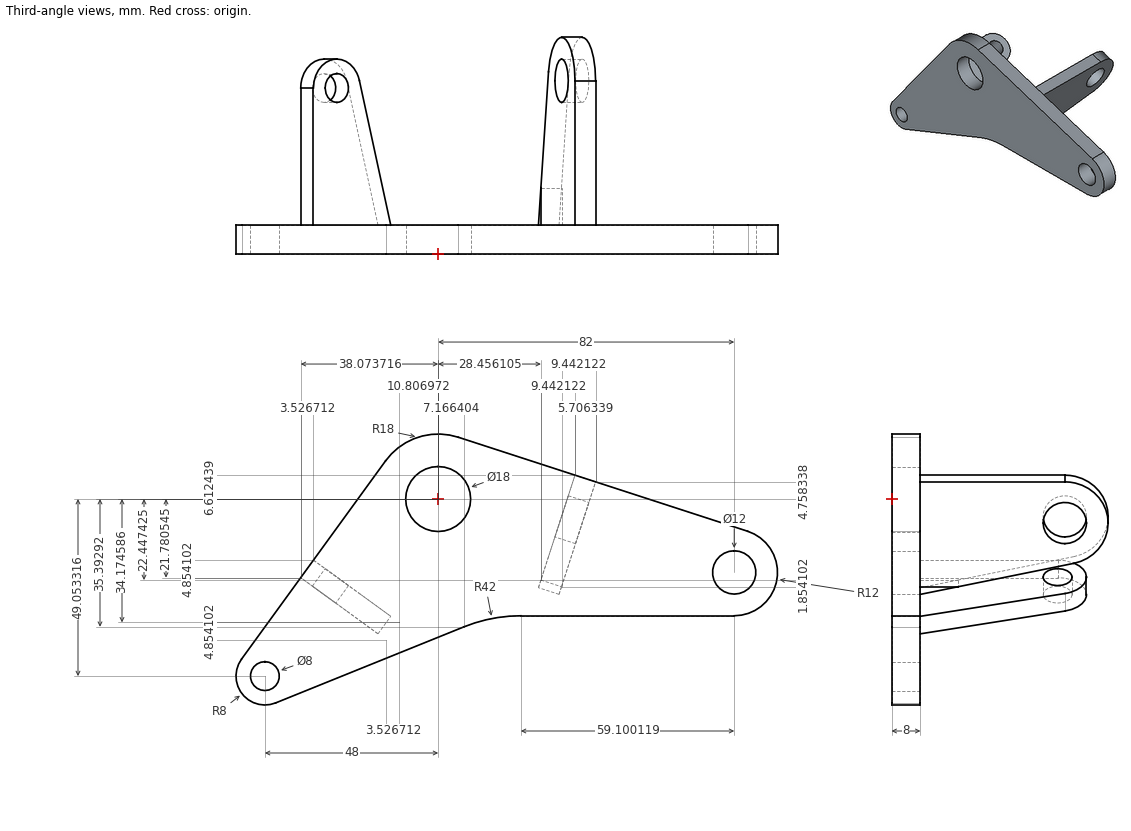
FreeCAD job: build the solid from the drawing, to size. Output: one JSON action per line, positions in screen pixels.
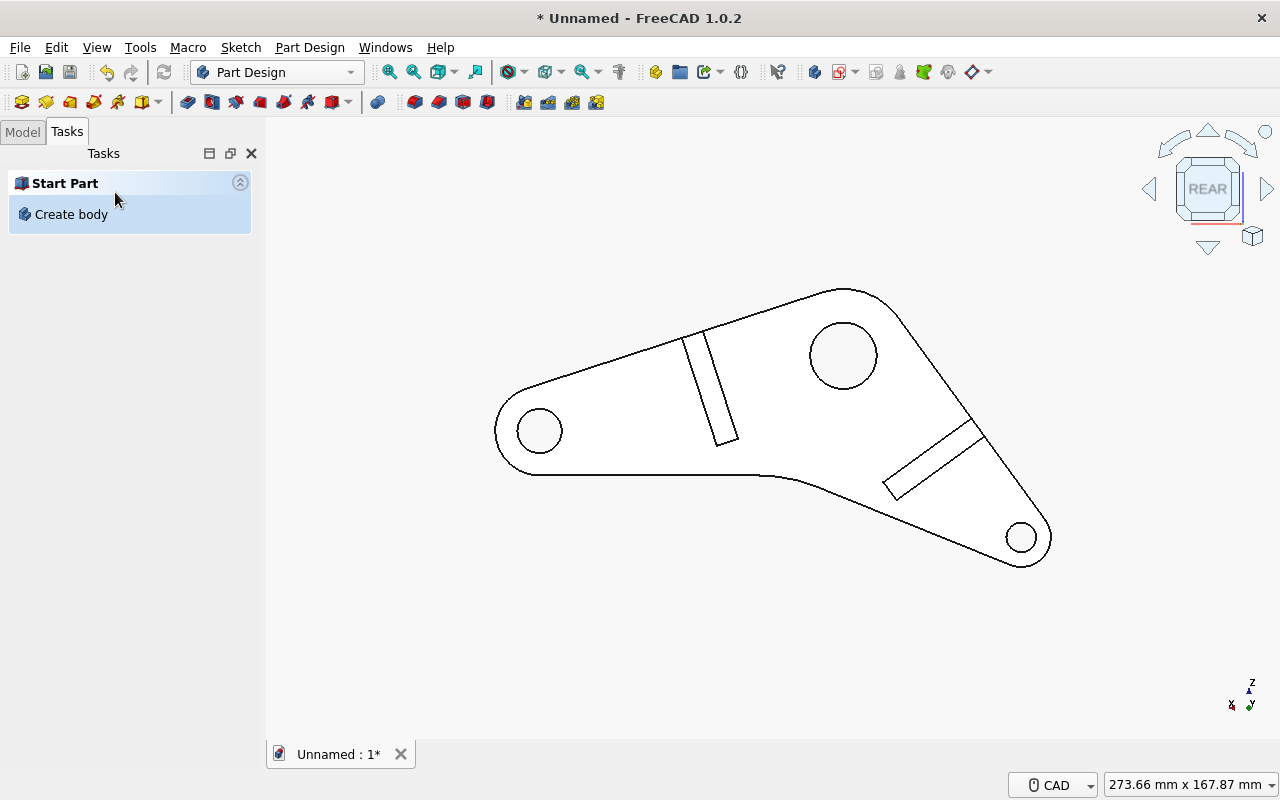
{"action": "key", "text": "5"}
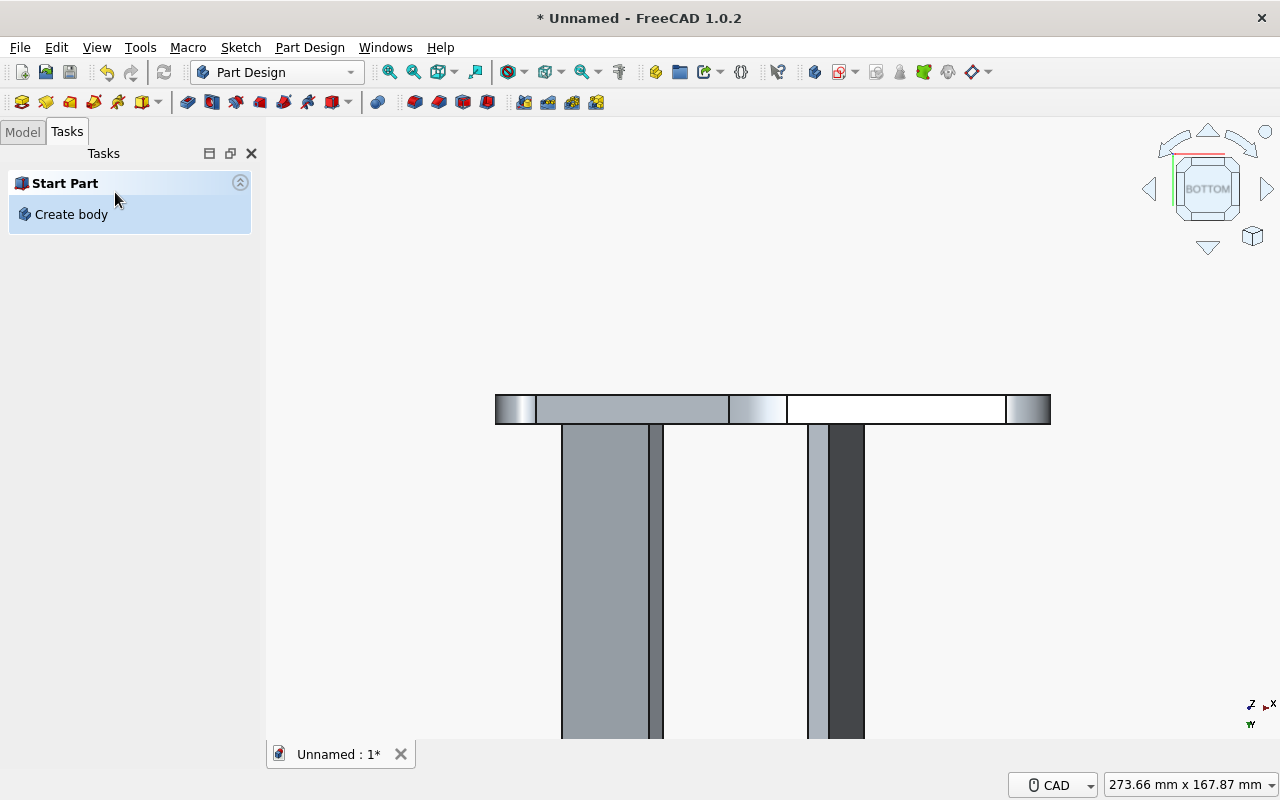
{"action": "key", "text": "v f"}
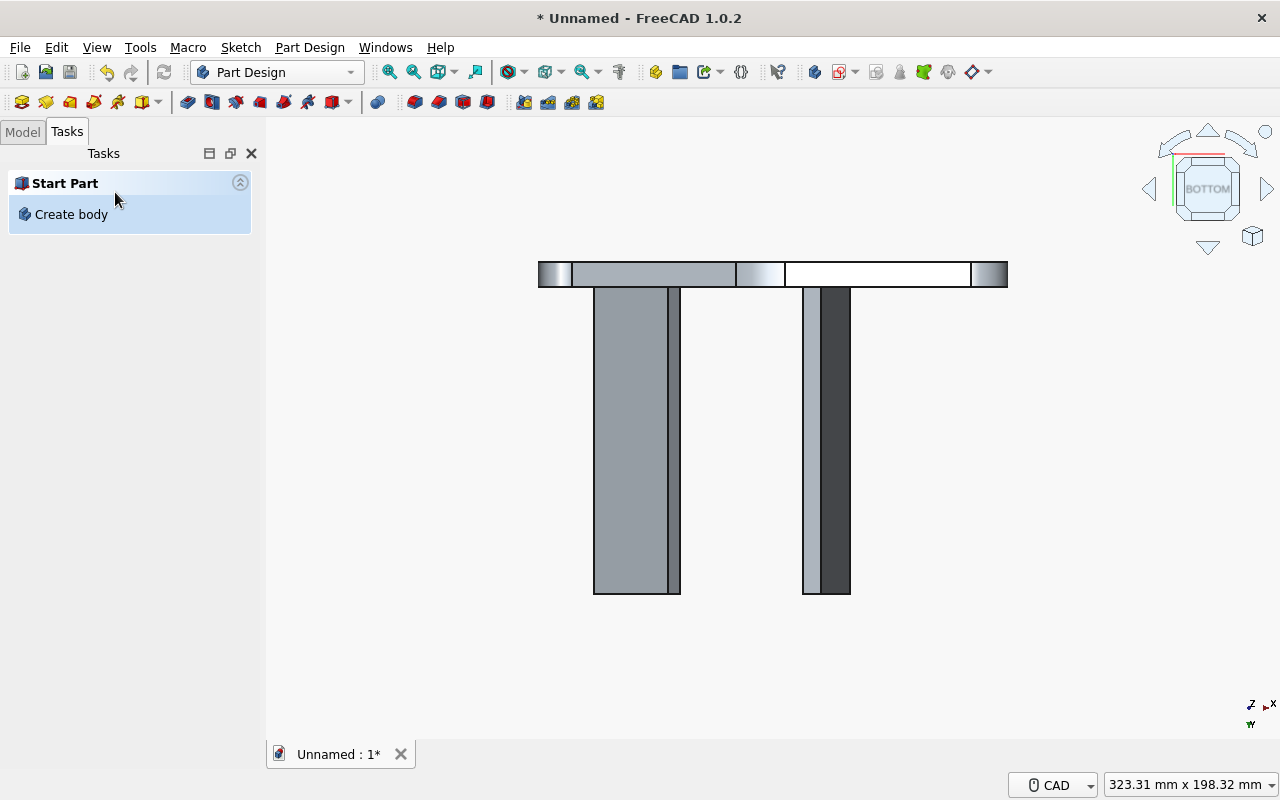
{"action": "left_click", "coordinate": [631, 527]}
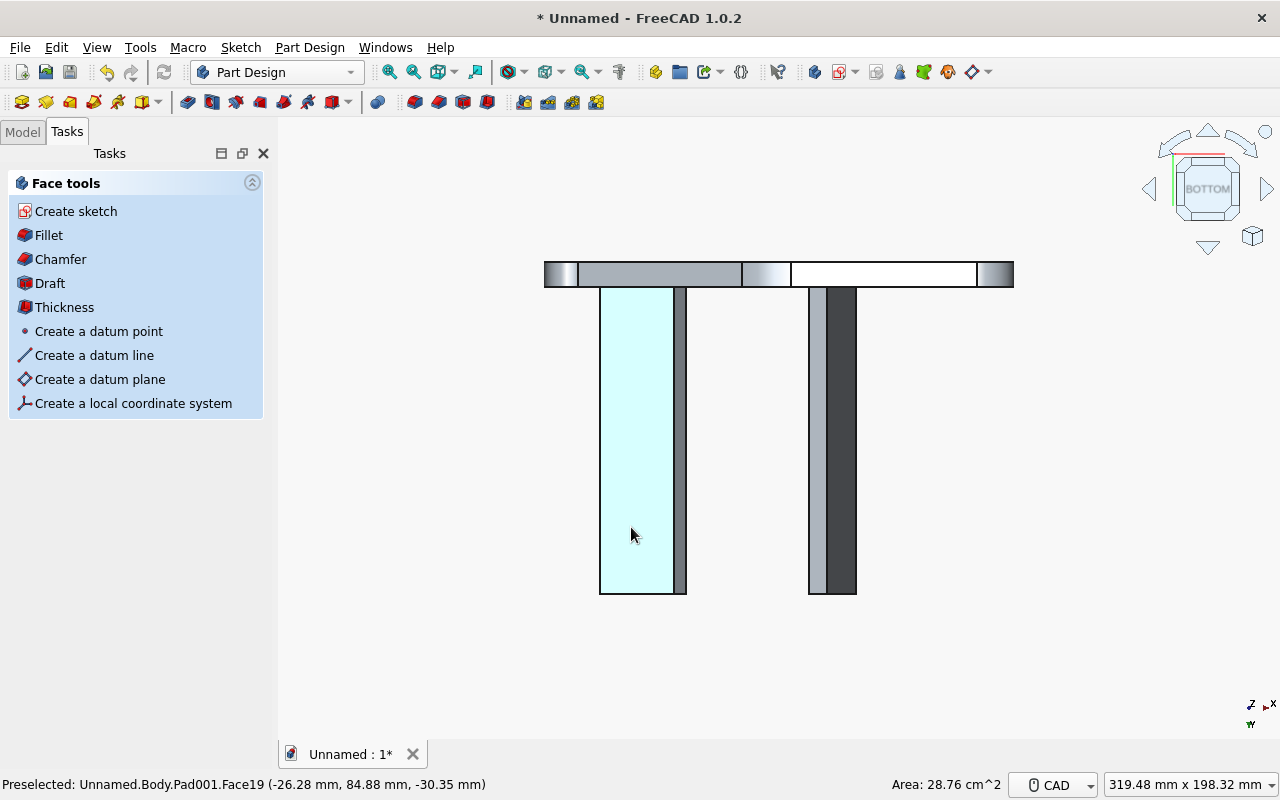
{"action": "left_click", "coordinate": [840, 72]}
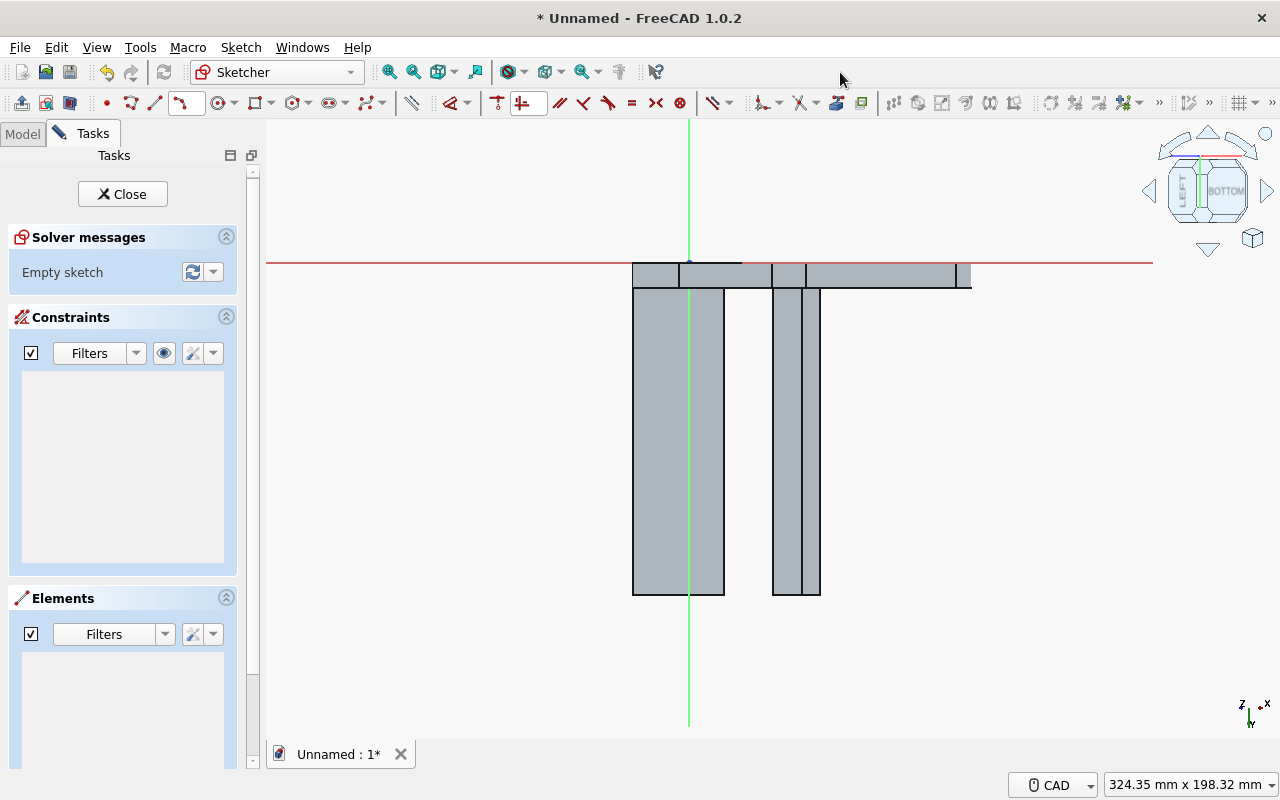
{"action": "left_click", "coordinate": [70, 104]}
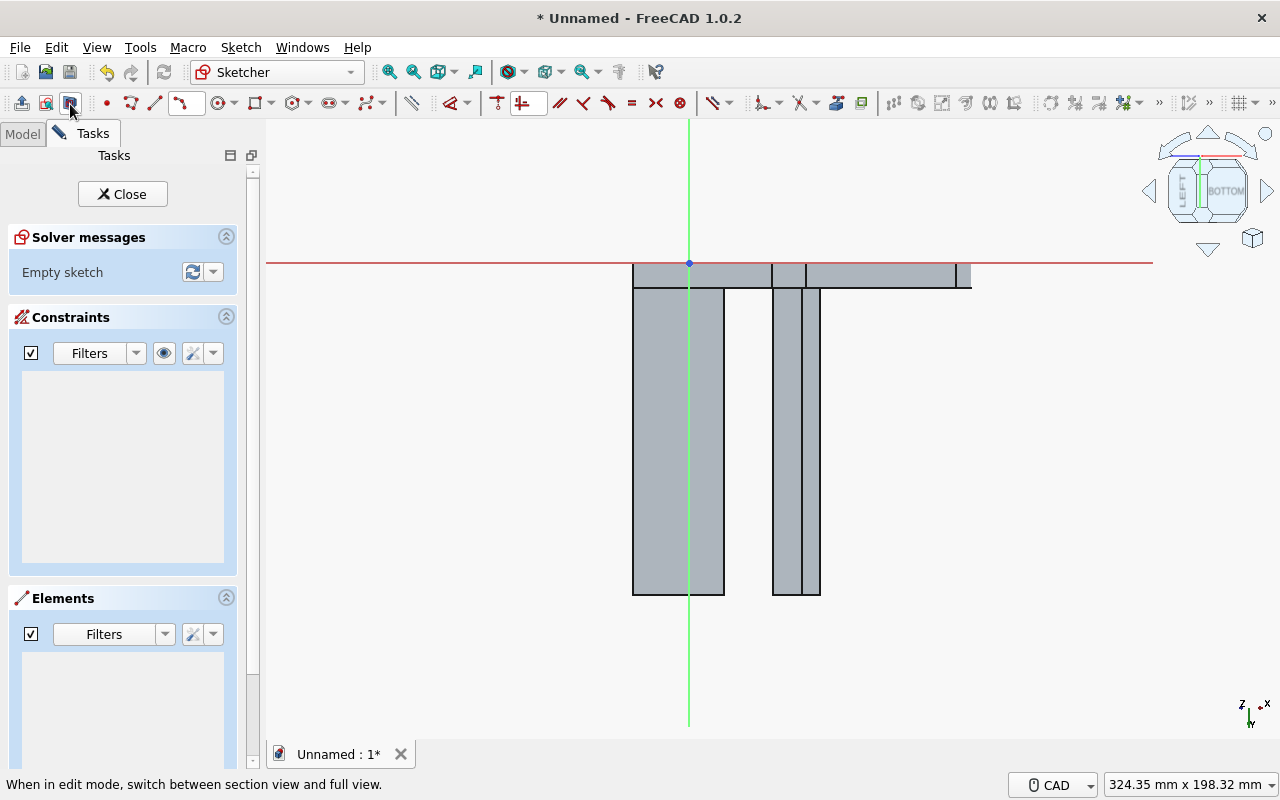
{"action": "left_click", "coordinate": [132, 104]}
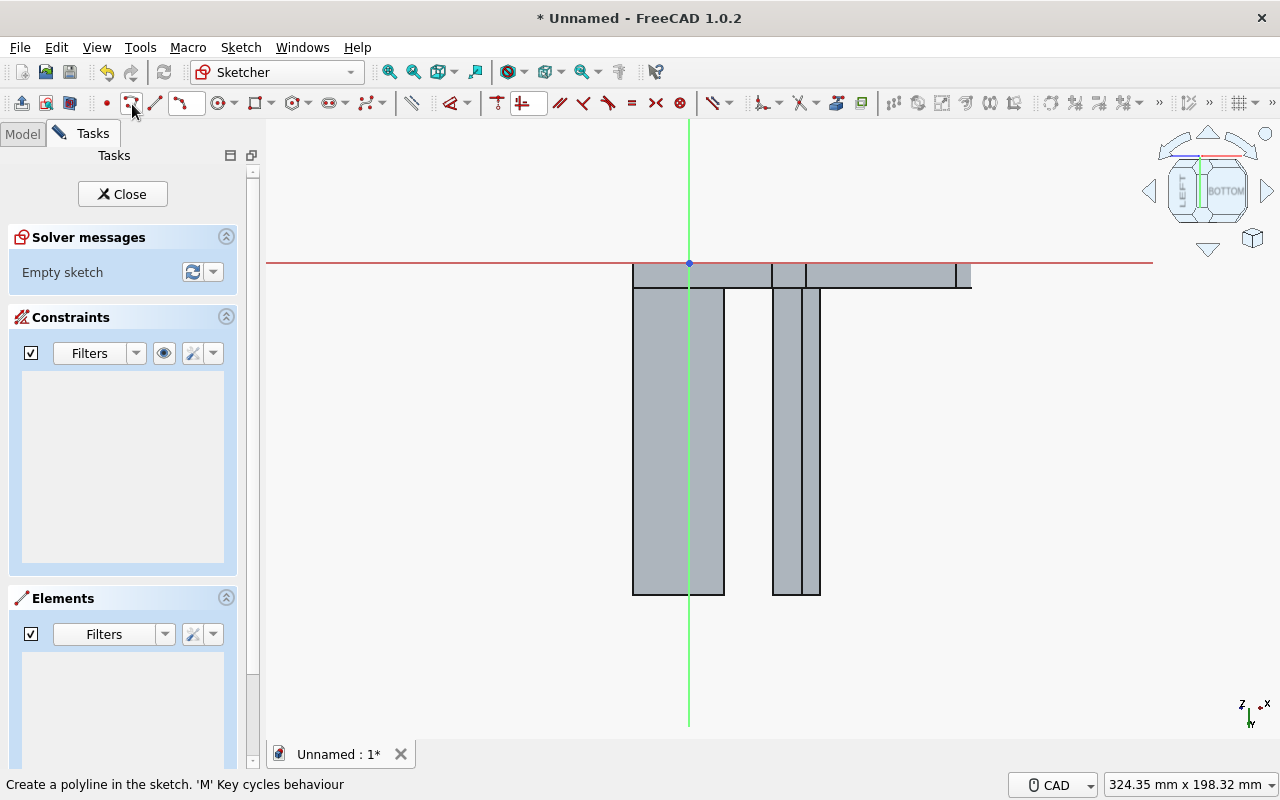
{"action": "left_click", "coordinate": [633, 407]}
{"action": "left_click", "coordinate": [614, 399]}
{"action": "left_click", "coordinate": [538, 609]}
{"action": "left_click", "coordinate": [746, 609]}
{"action": "left_click", "coordinate": [730, 288]}
{"action": "left_click", "coordinate": [715, 288]}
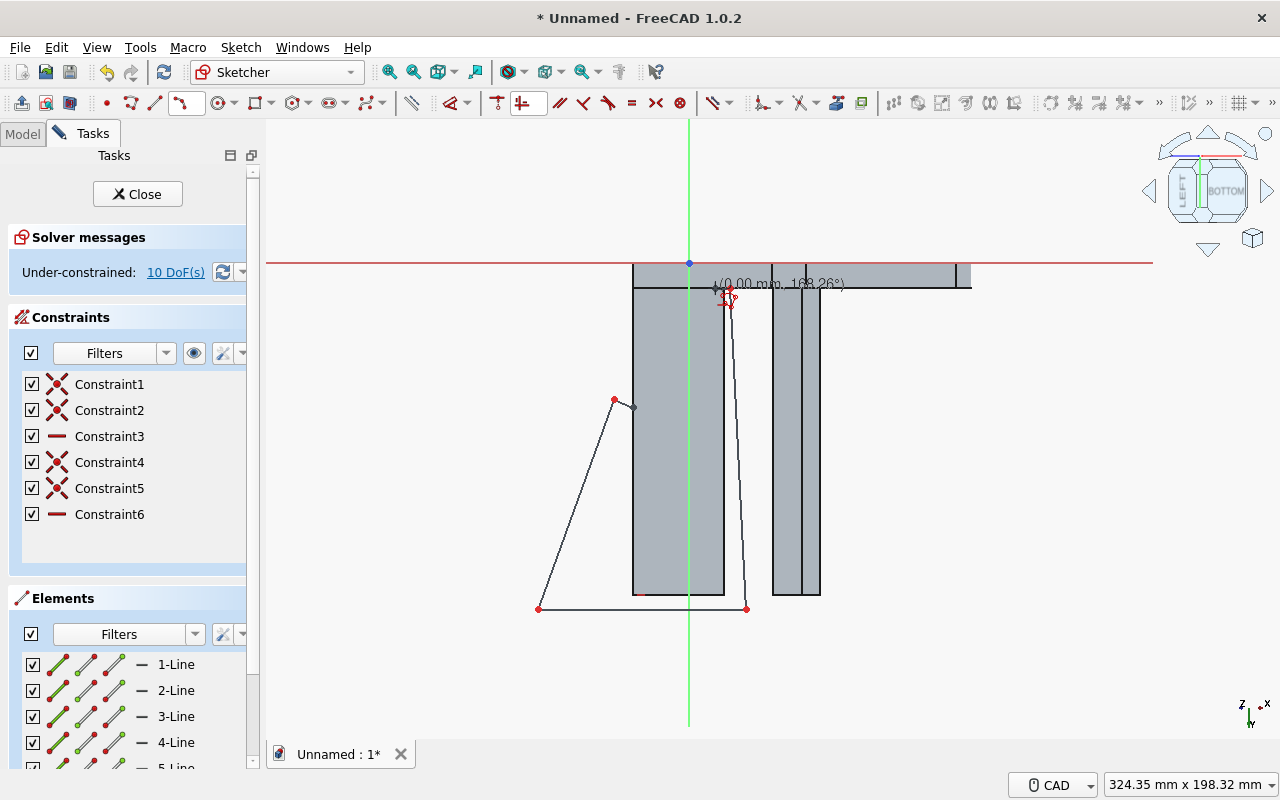
{"action": "scroll", "coordinate": [682, 414], "scroll_direction": "up", "scroll_amount": 5}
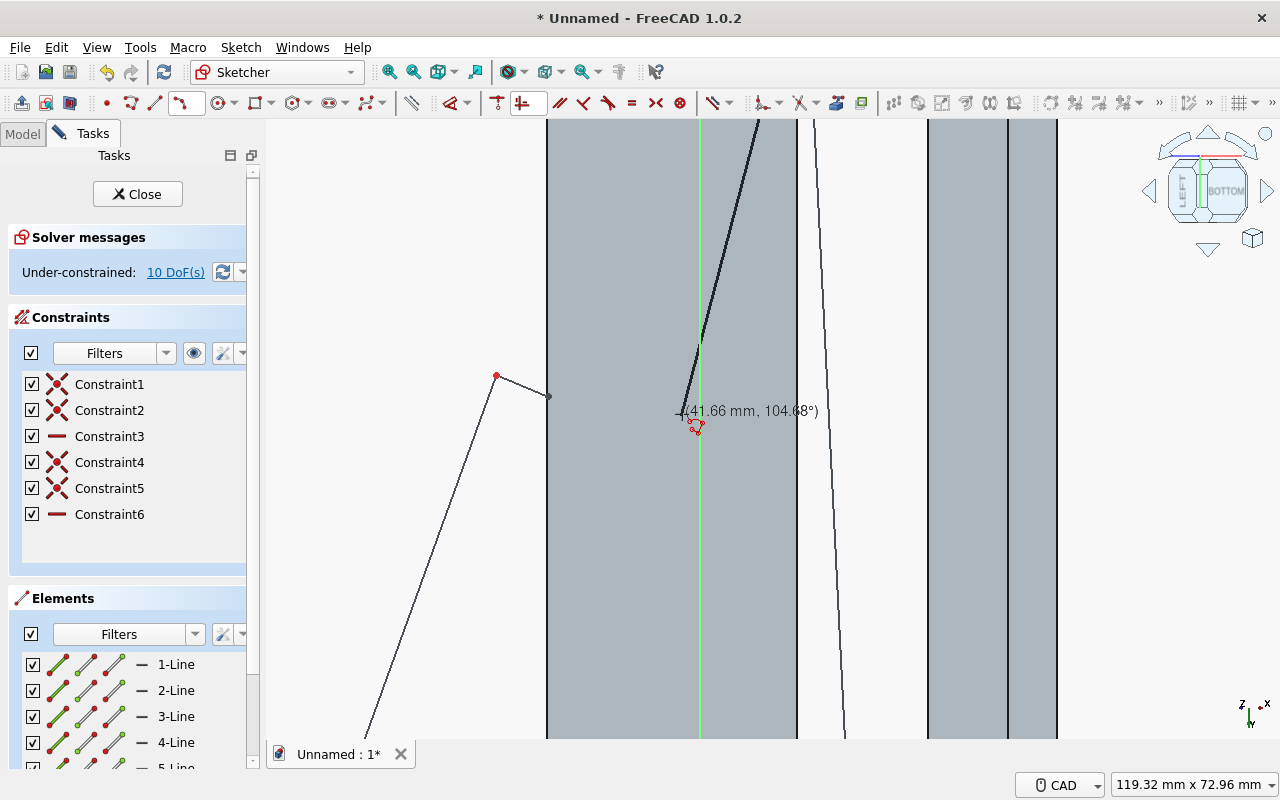
{"action": "left_click", "coordinate": [681, 412]}
{"action": "right_click", "coordinate": [681, 412]}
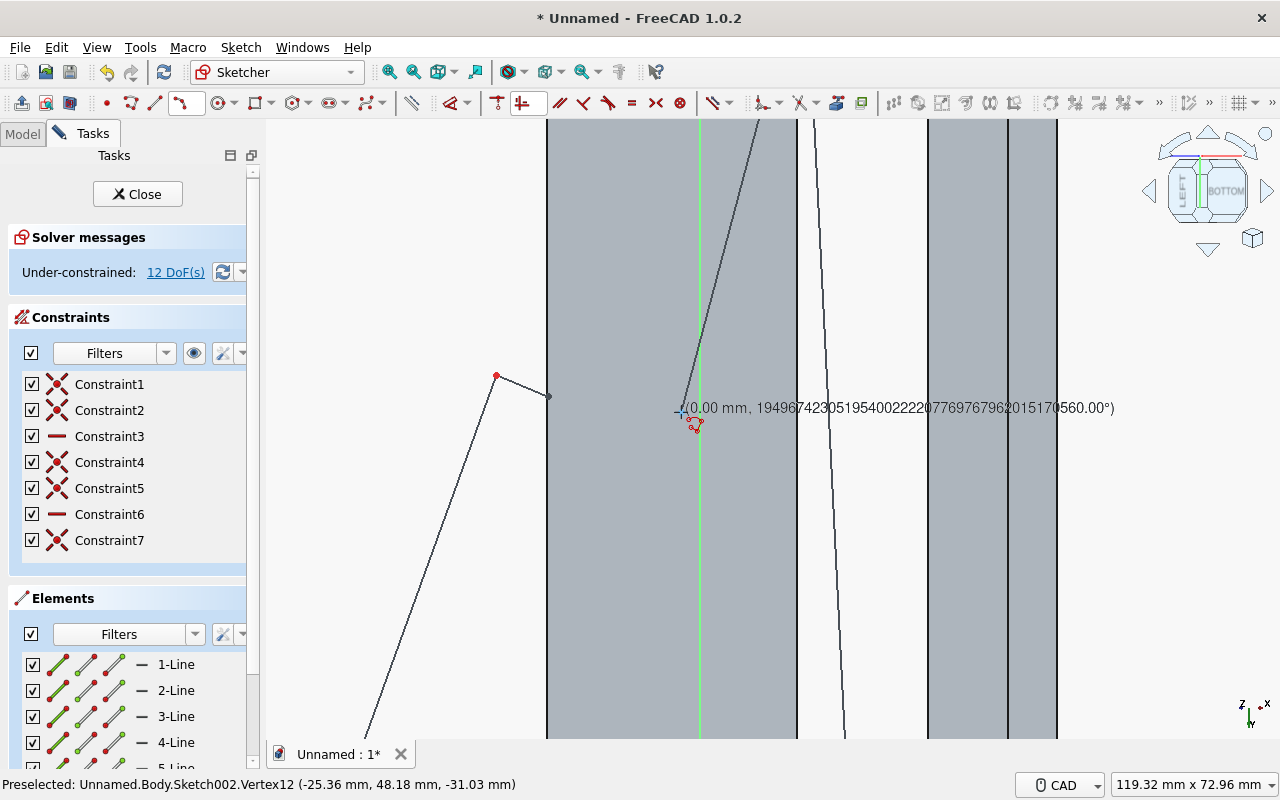
{"action": "left_click", "coordinate": [180, 104]}